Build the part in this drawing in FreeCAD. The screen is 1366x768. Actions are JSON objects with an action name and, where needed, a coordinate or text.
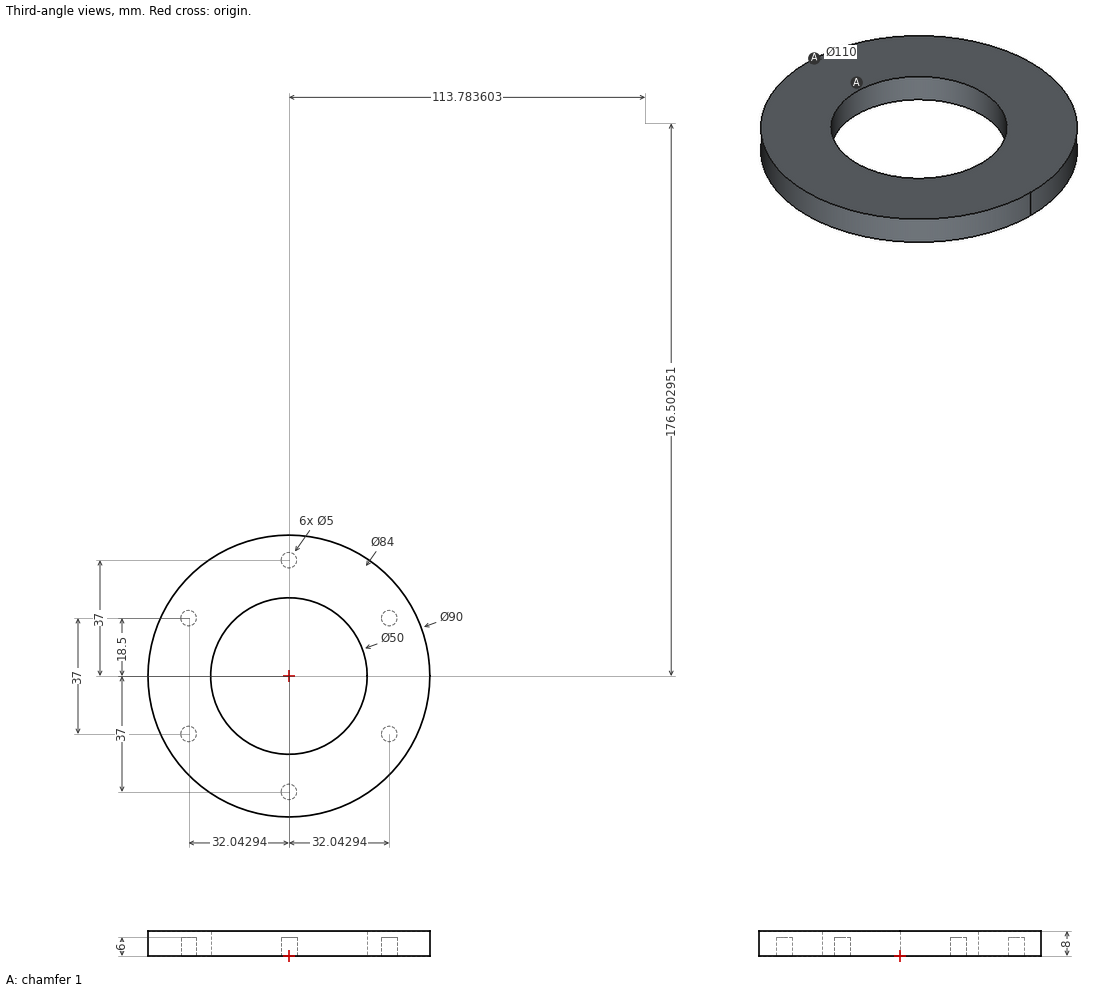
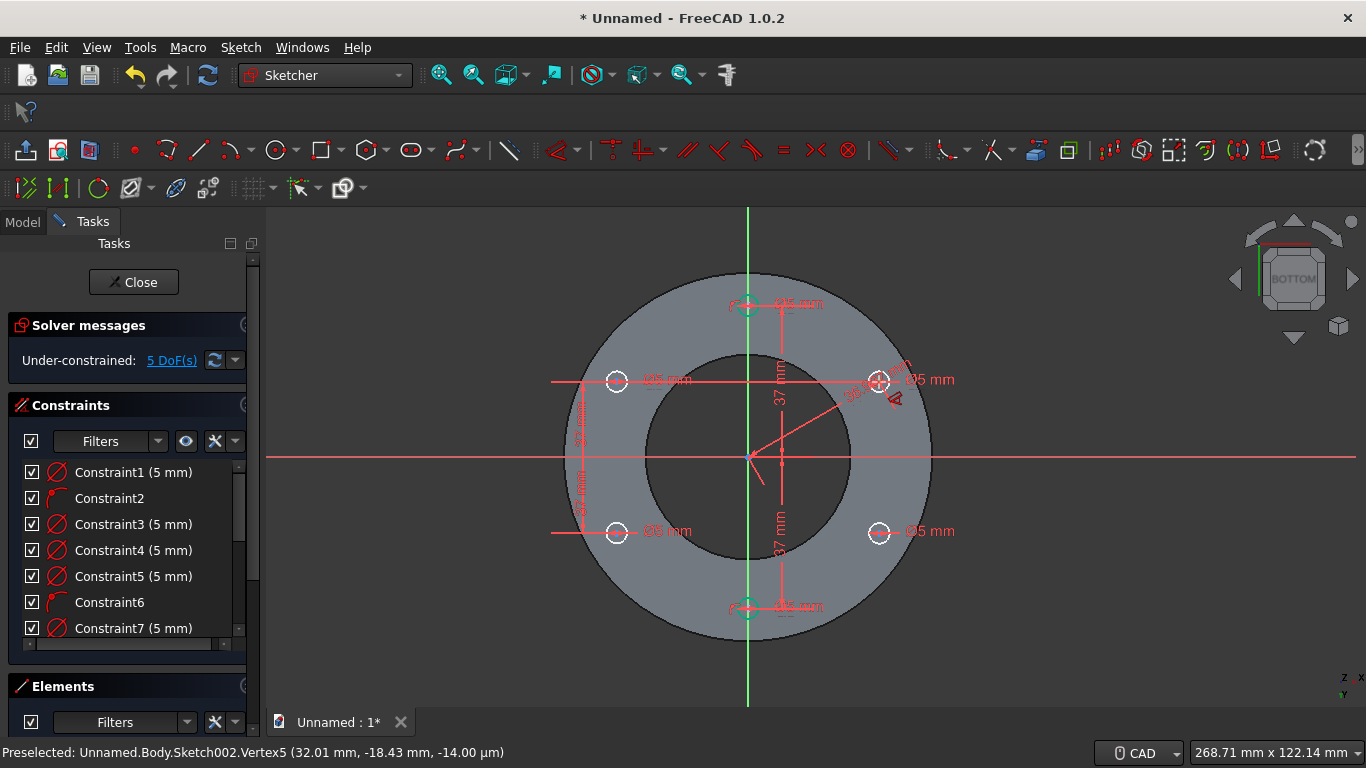
{"action": "left_click", "coordinate": [879, 533]}
{"action": "left_click", "coordinate": [913, 423]}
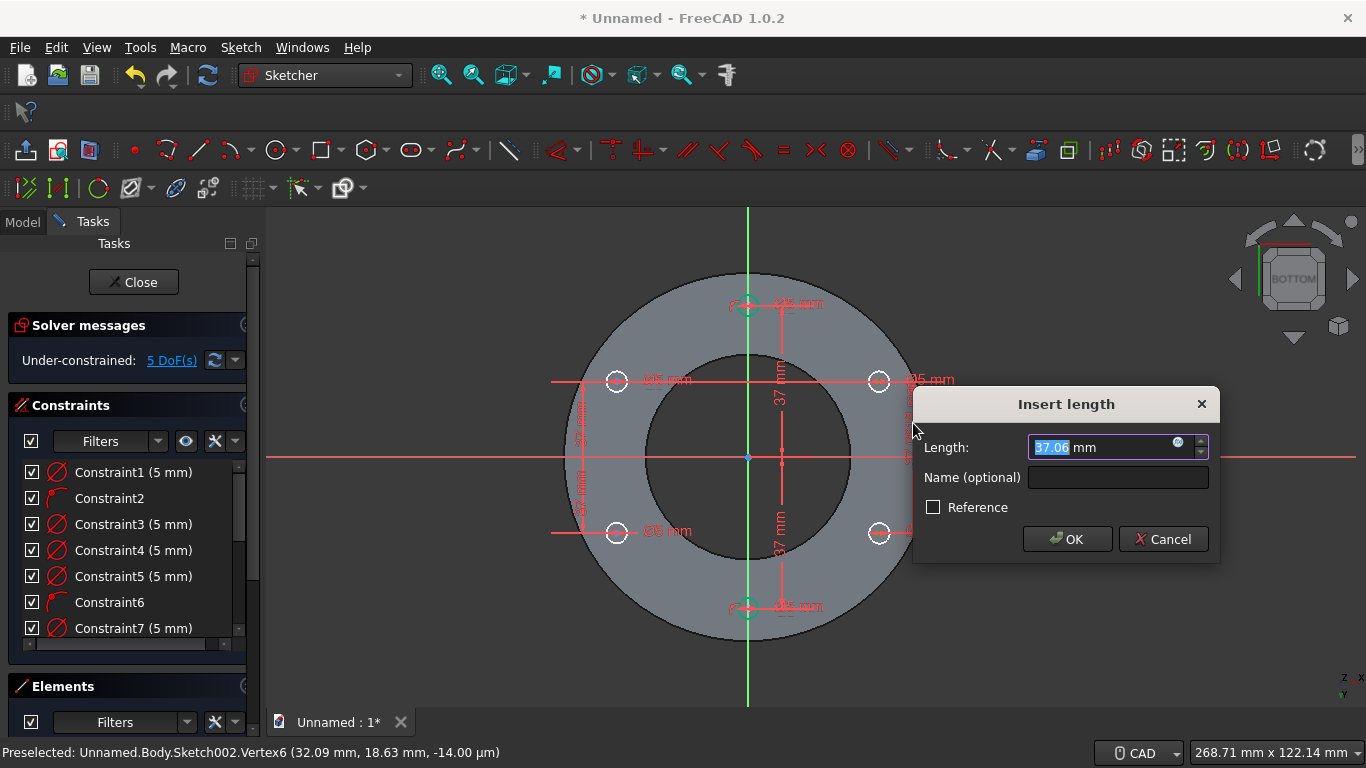
{"action": "type", "text": "37"}
{"action": "key", "text": "Return"}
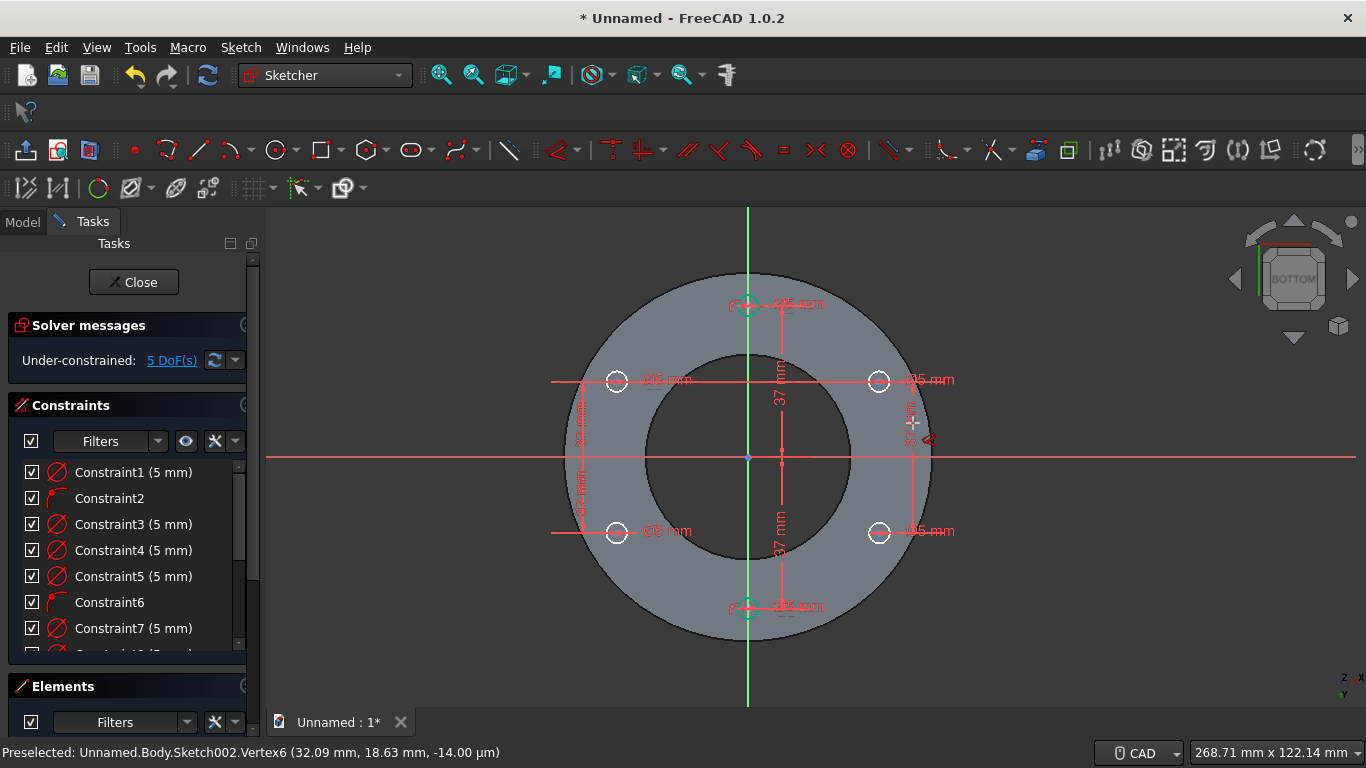
{"action": "left_click", "coordinate": [617, 533]}
{"action": "left_click", "coordinate": [583, 513]}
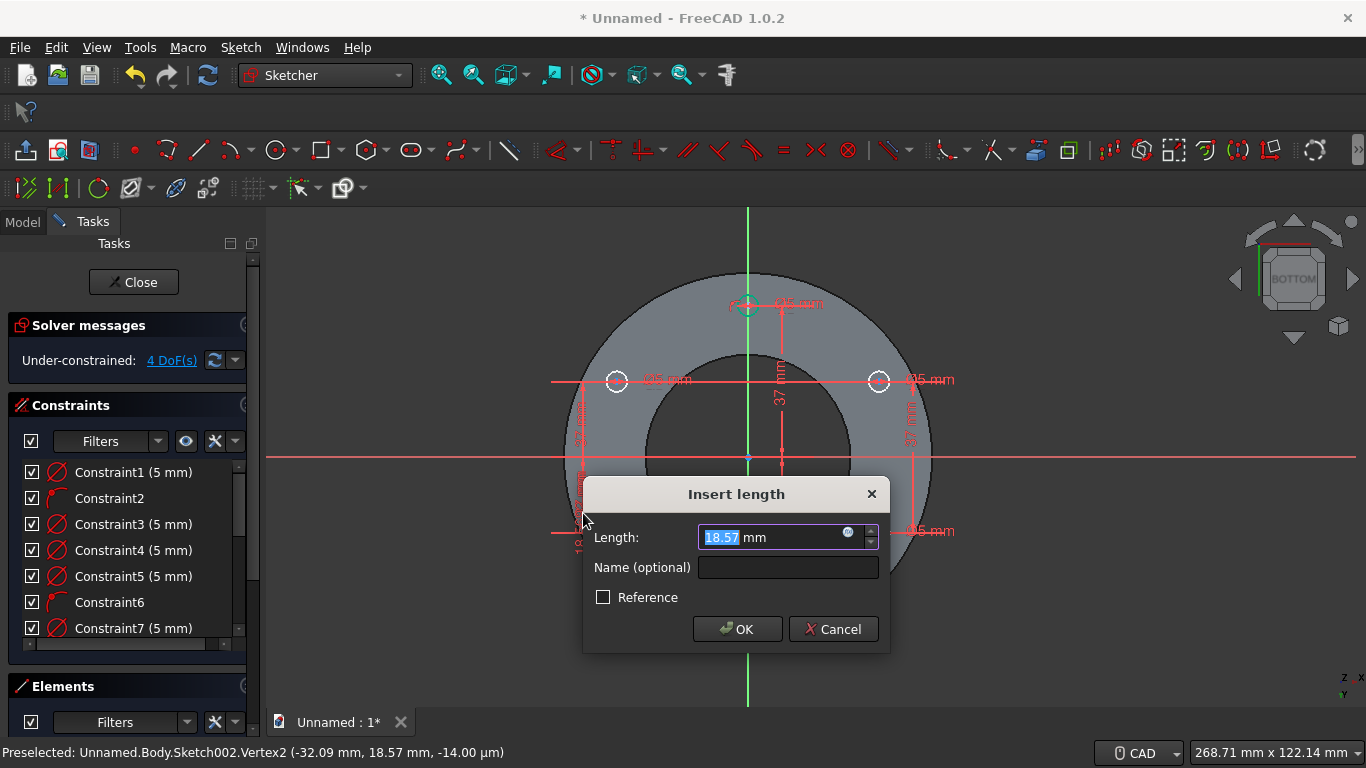
{"action": "type", "text": "18.5"}
{"action": "key", "text": "Return"}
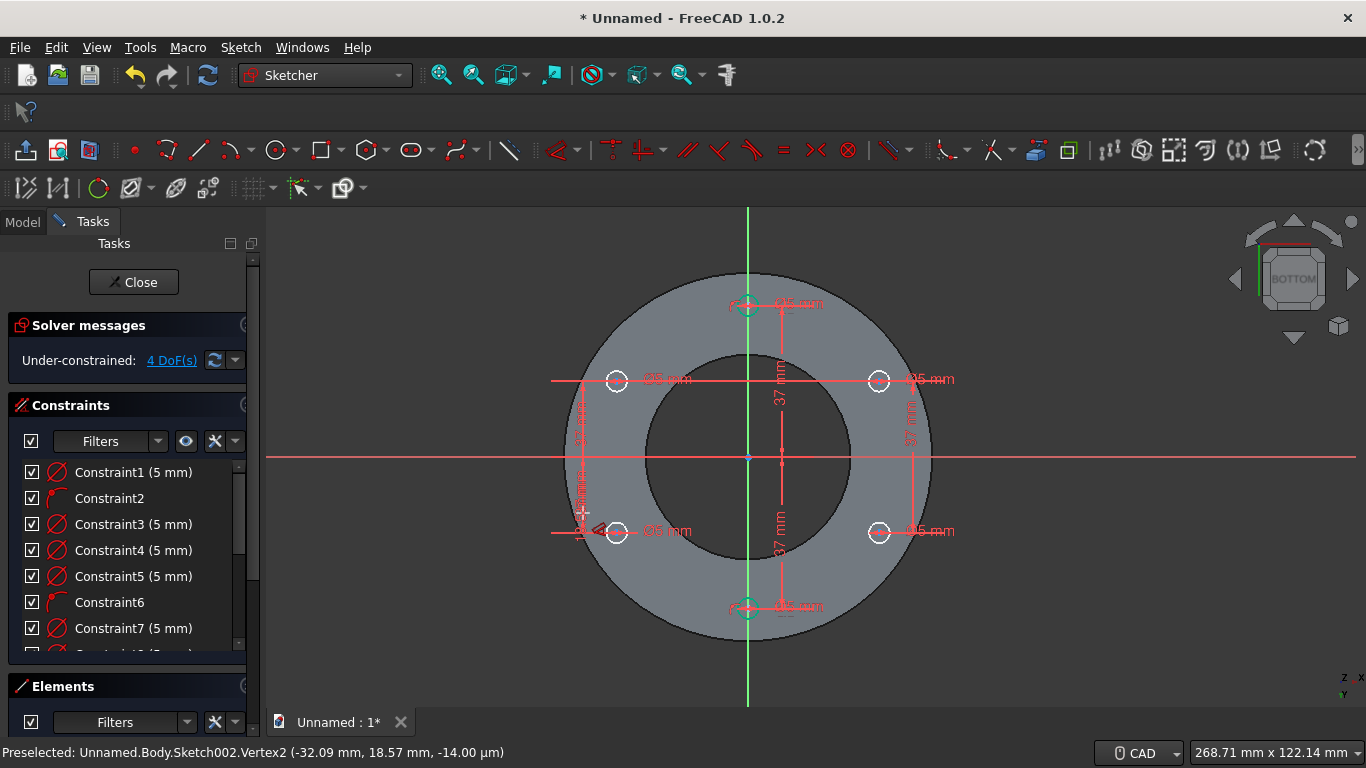
{"action": "left_click", "coordinate": [617, 533]}
{"action": "left_click", "coordinate": [682, 567]}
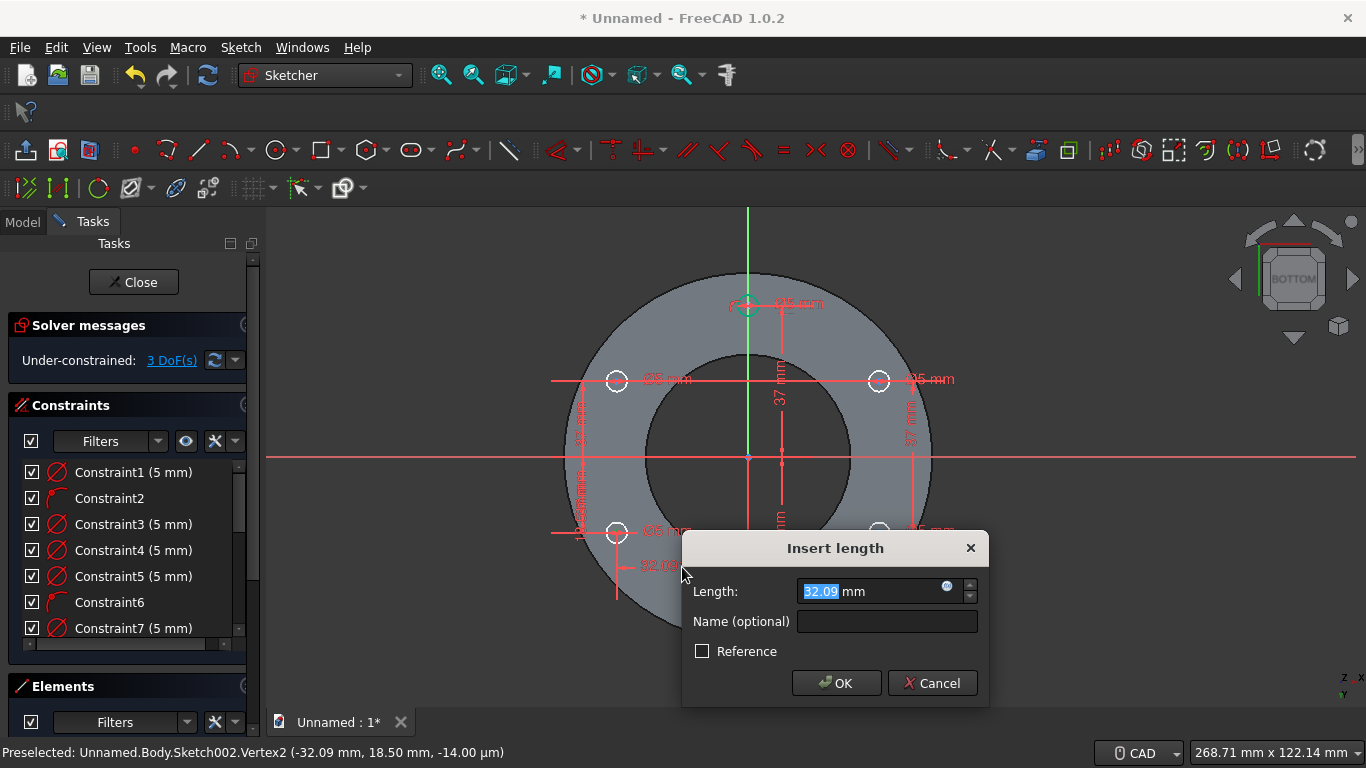
{"action": "type", "text": "32.04294"}
{"action": "key", "text": "Return"}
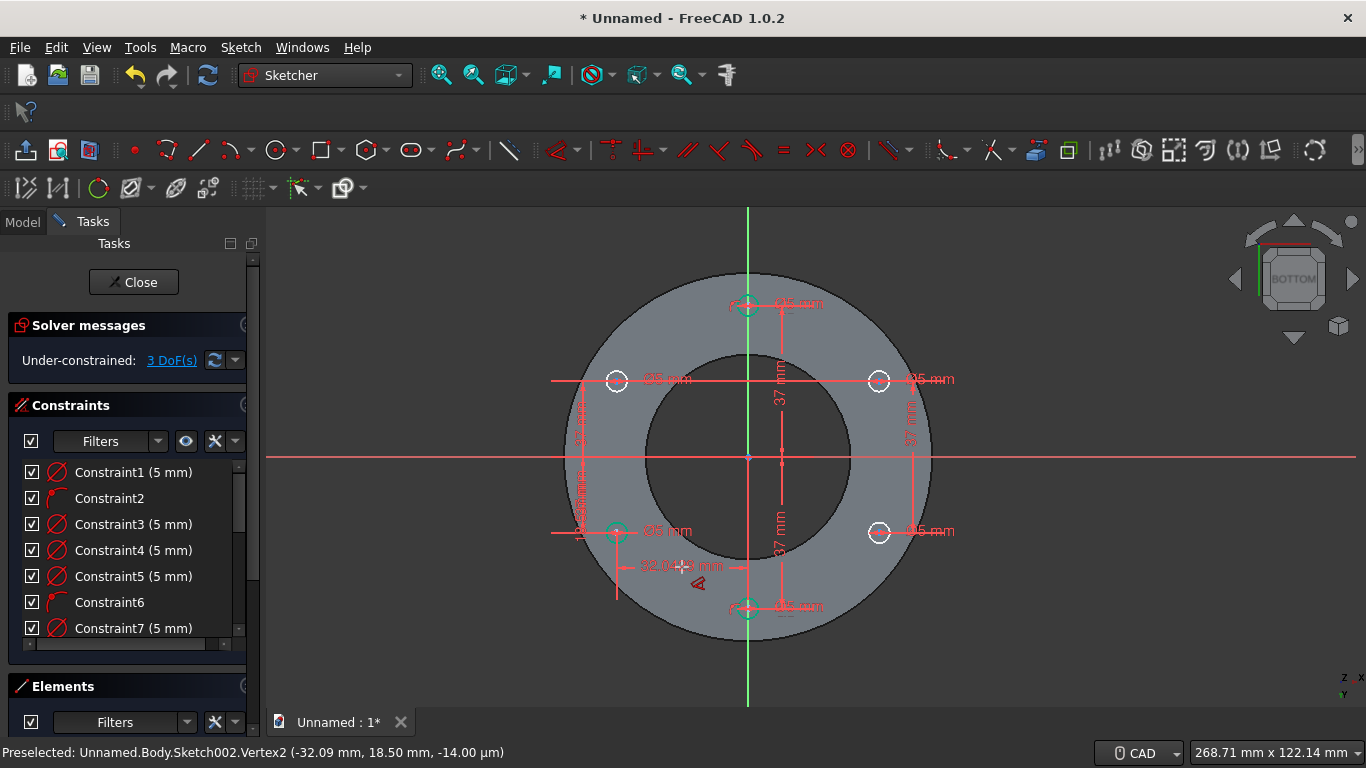
{"action": "left_click", "coordinate": [617, 381]}
{"action": "left_click", "coordinate": [682, 347]}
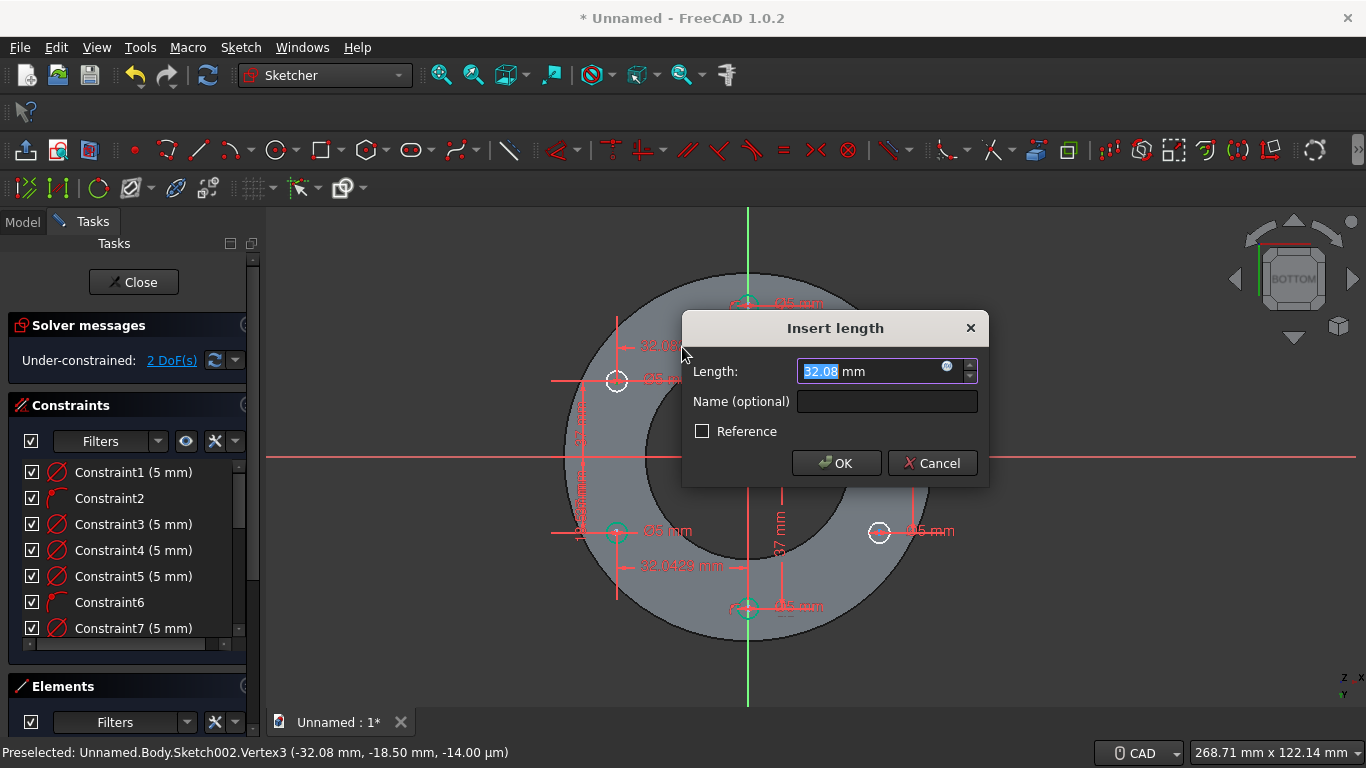
{"action": "type", "text": "32.04294"}
{"action": "key", "text": "Return"}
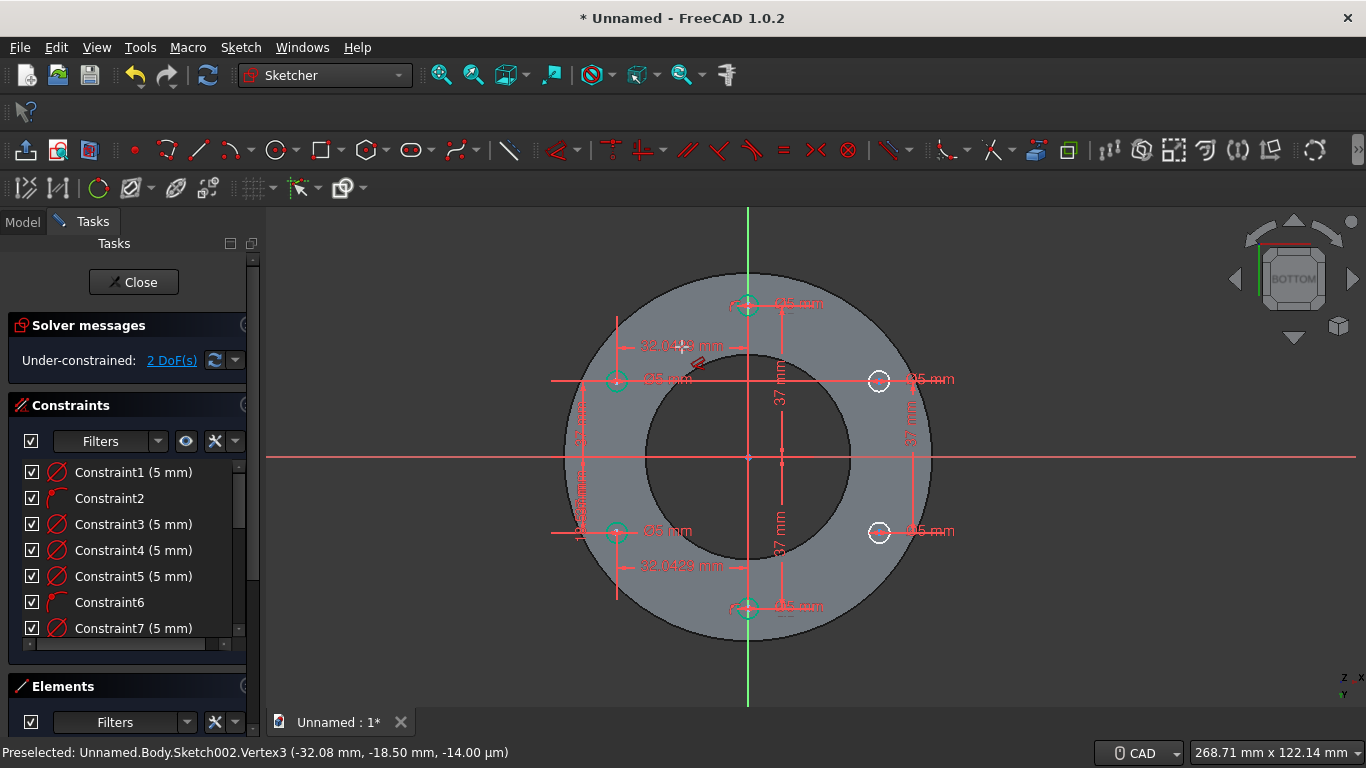
{"action": "left_click", "coordinate": [879, 381]}
{"action": "left_click", "coordinate": [814, 347]}